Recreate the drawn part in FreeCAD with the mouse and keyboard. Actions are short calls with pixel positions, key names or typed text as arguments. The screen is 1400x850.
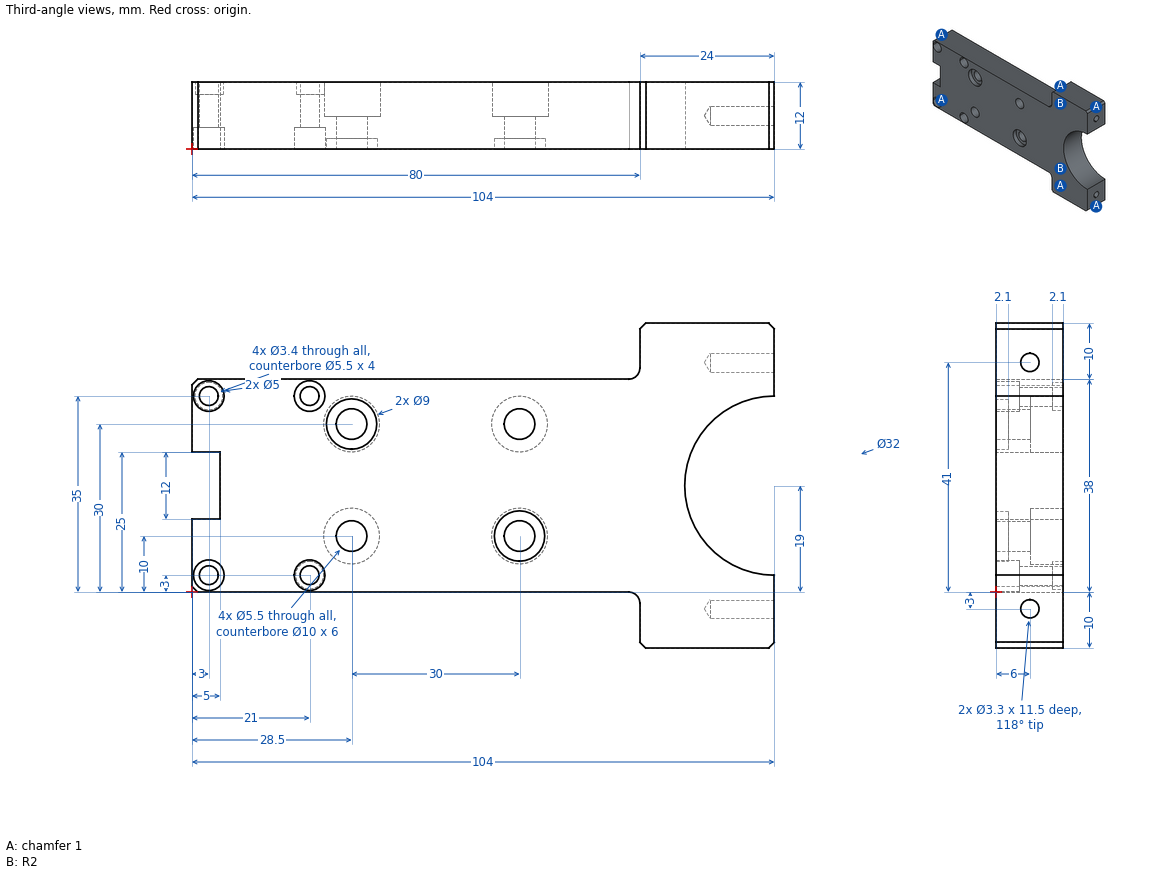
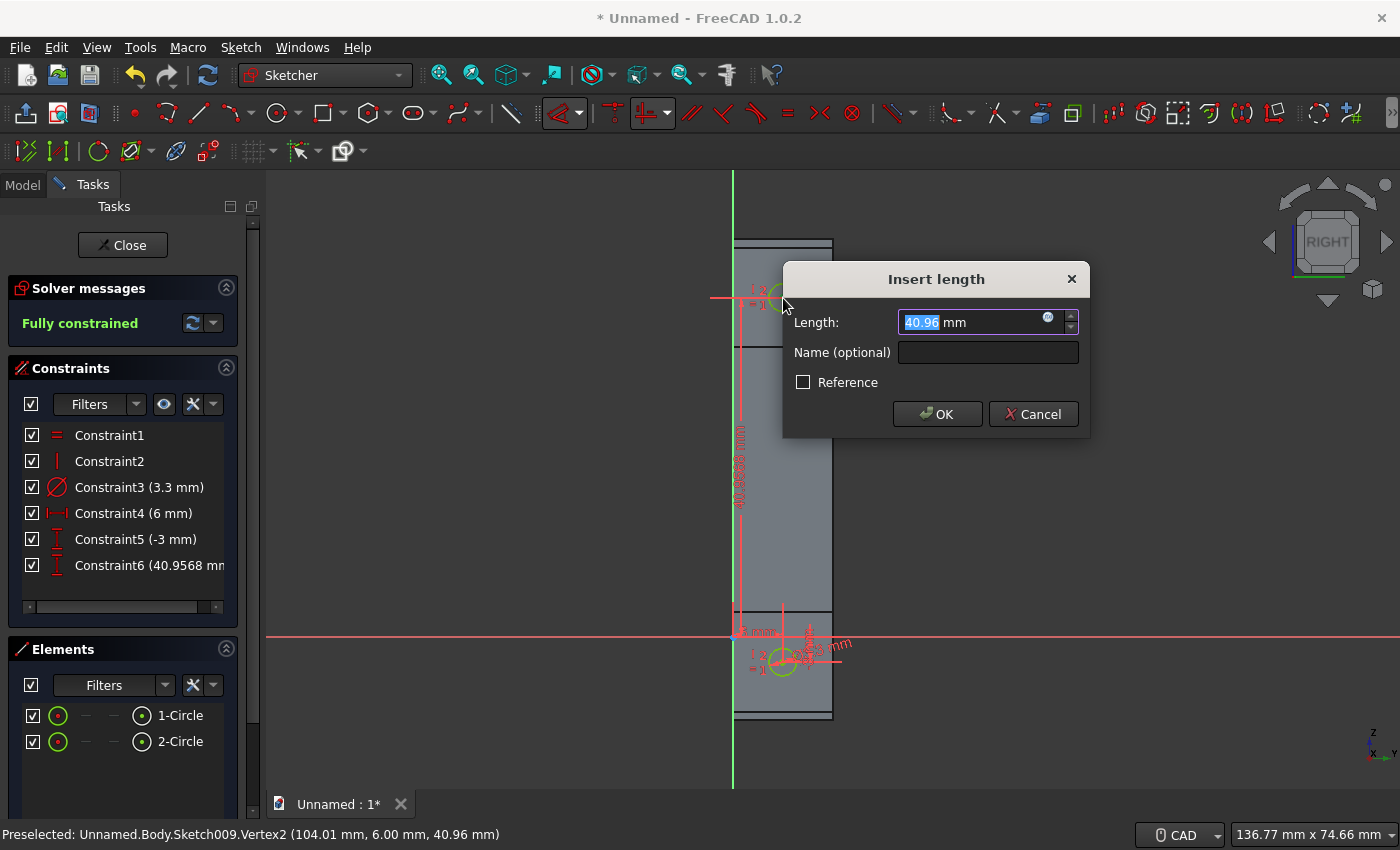
text(41)
key(Return)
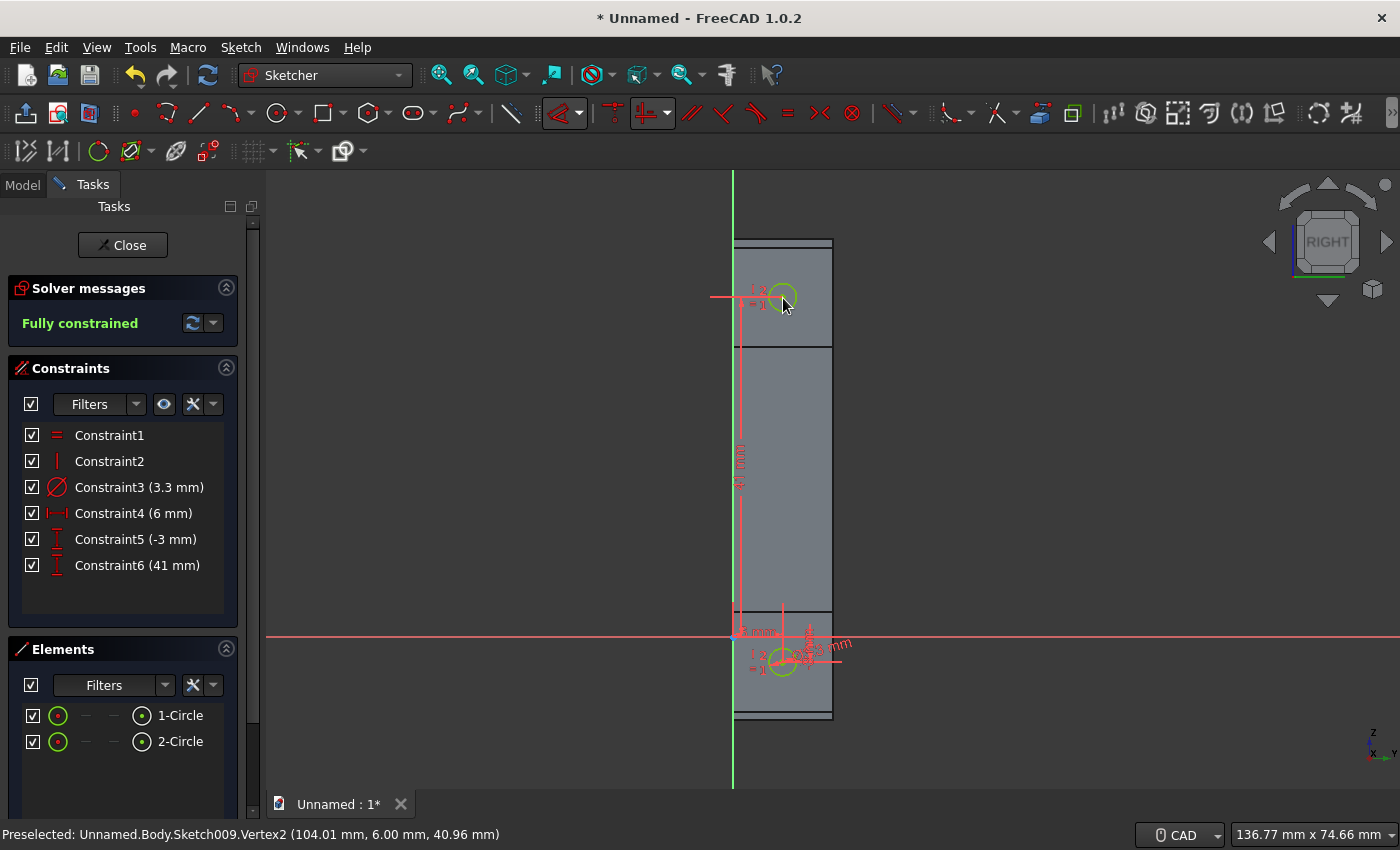
click(123, 245)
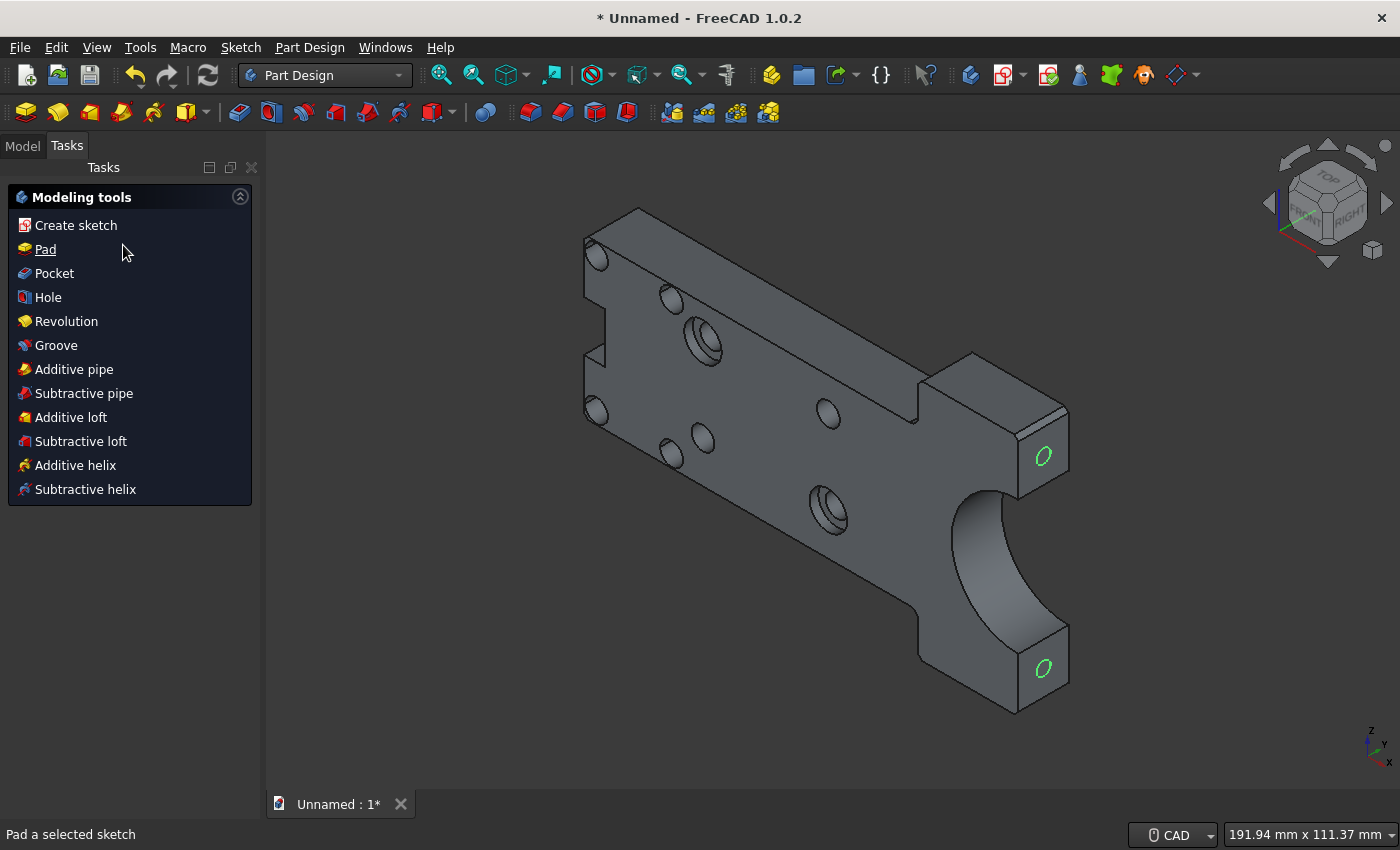
click(272, 112)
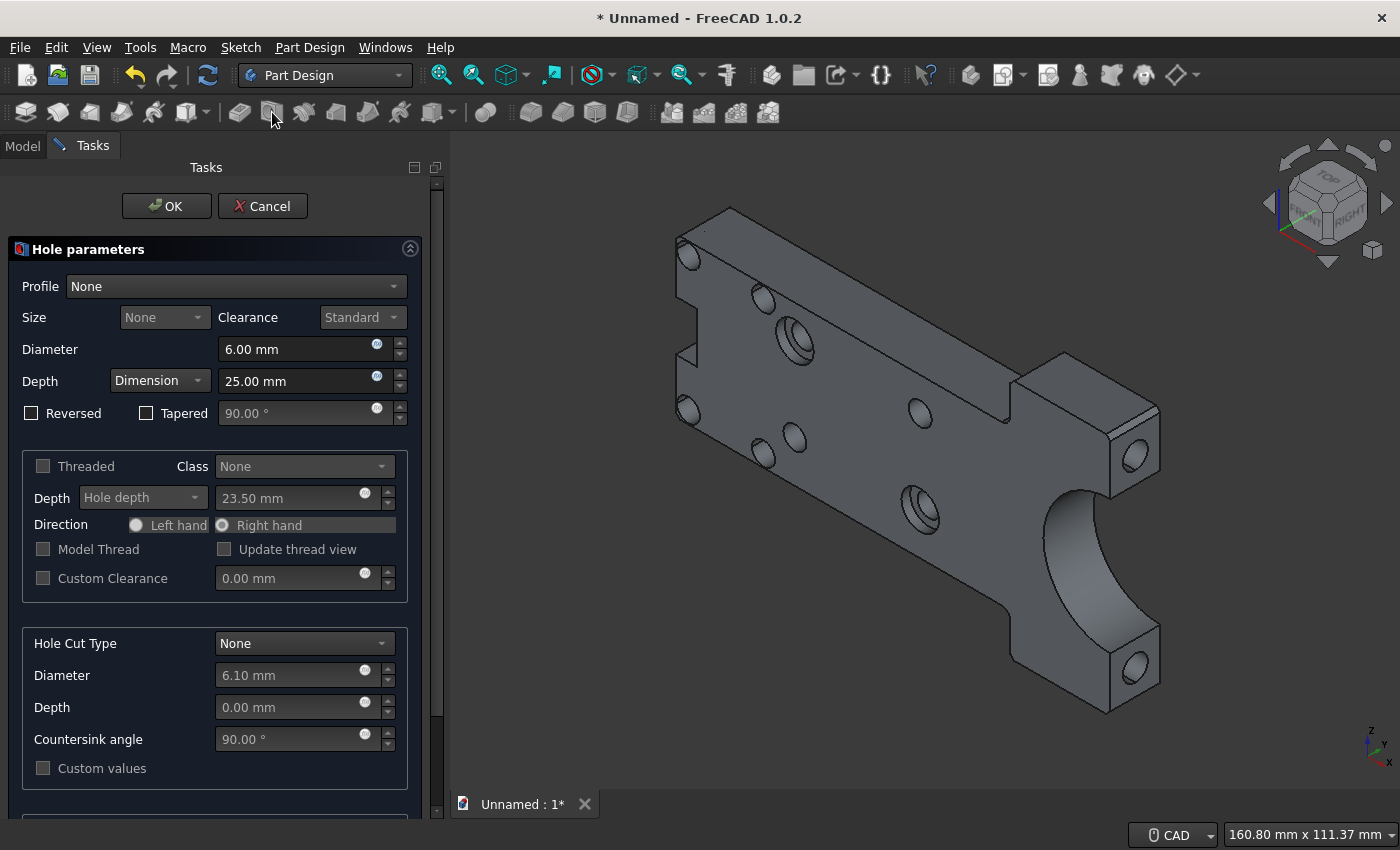
triple_click(305, 349)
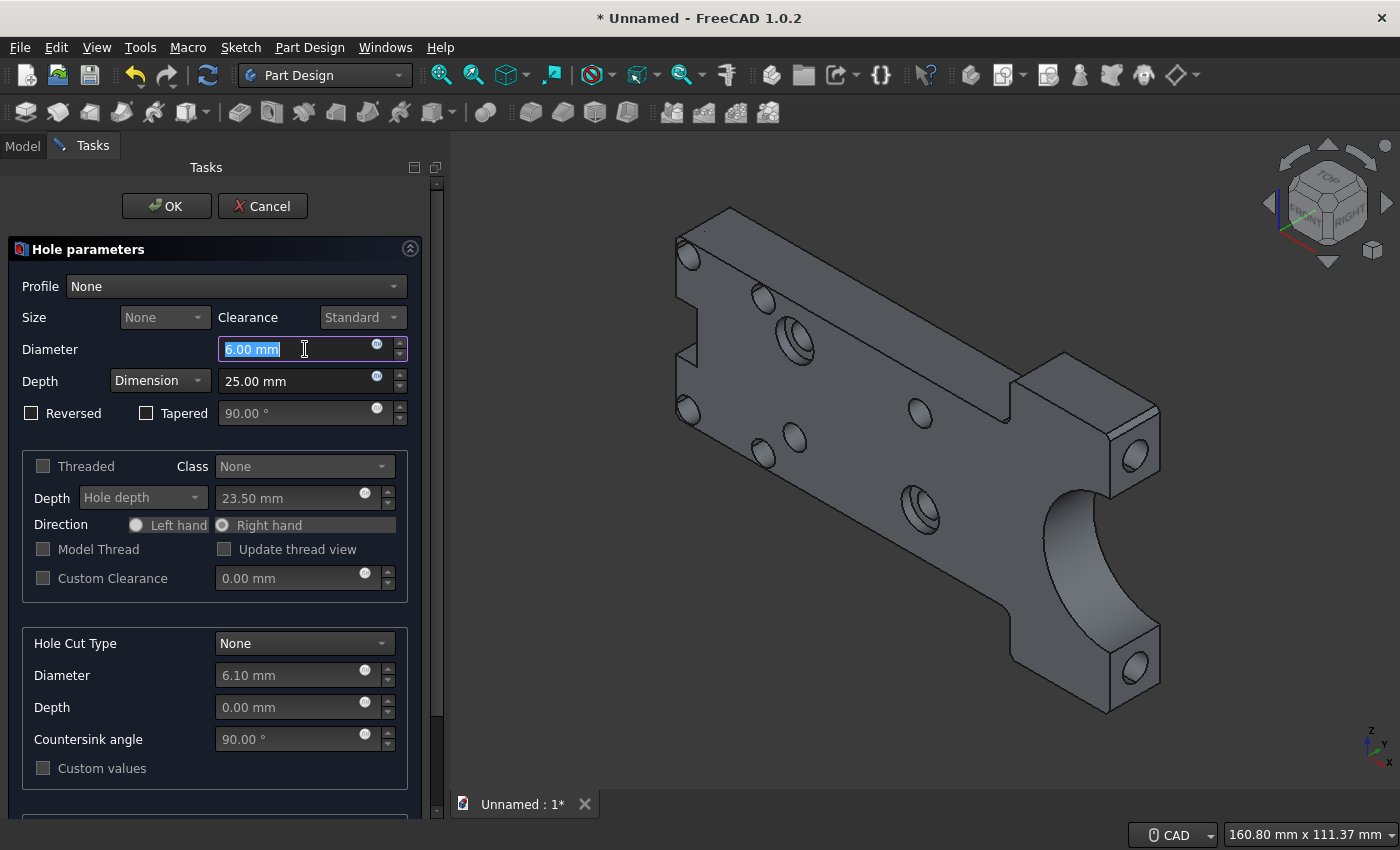
text(3.3)
key(Tab)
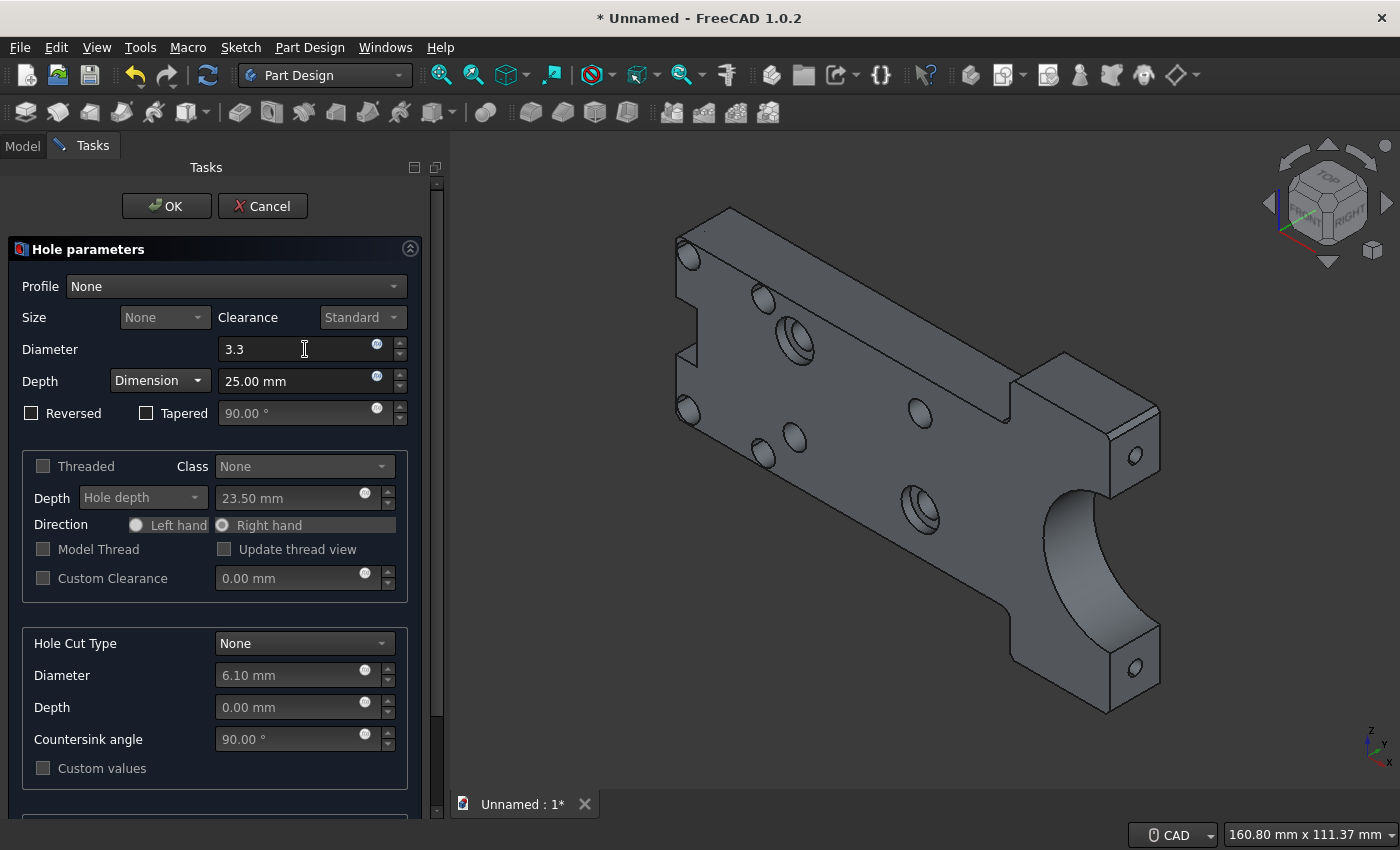
triple_click(305, 381)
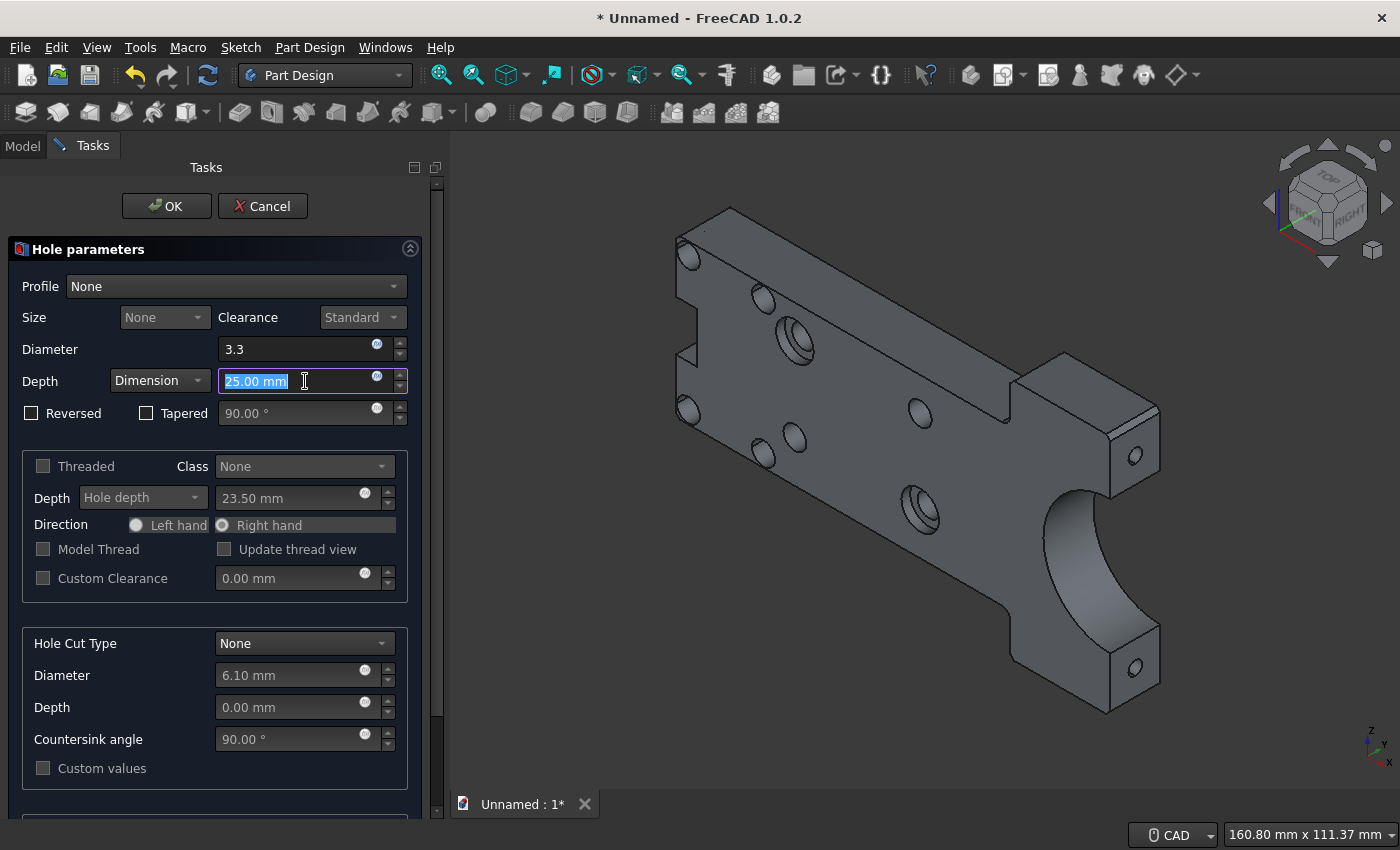
text(11.5)
key(Tab)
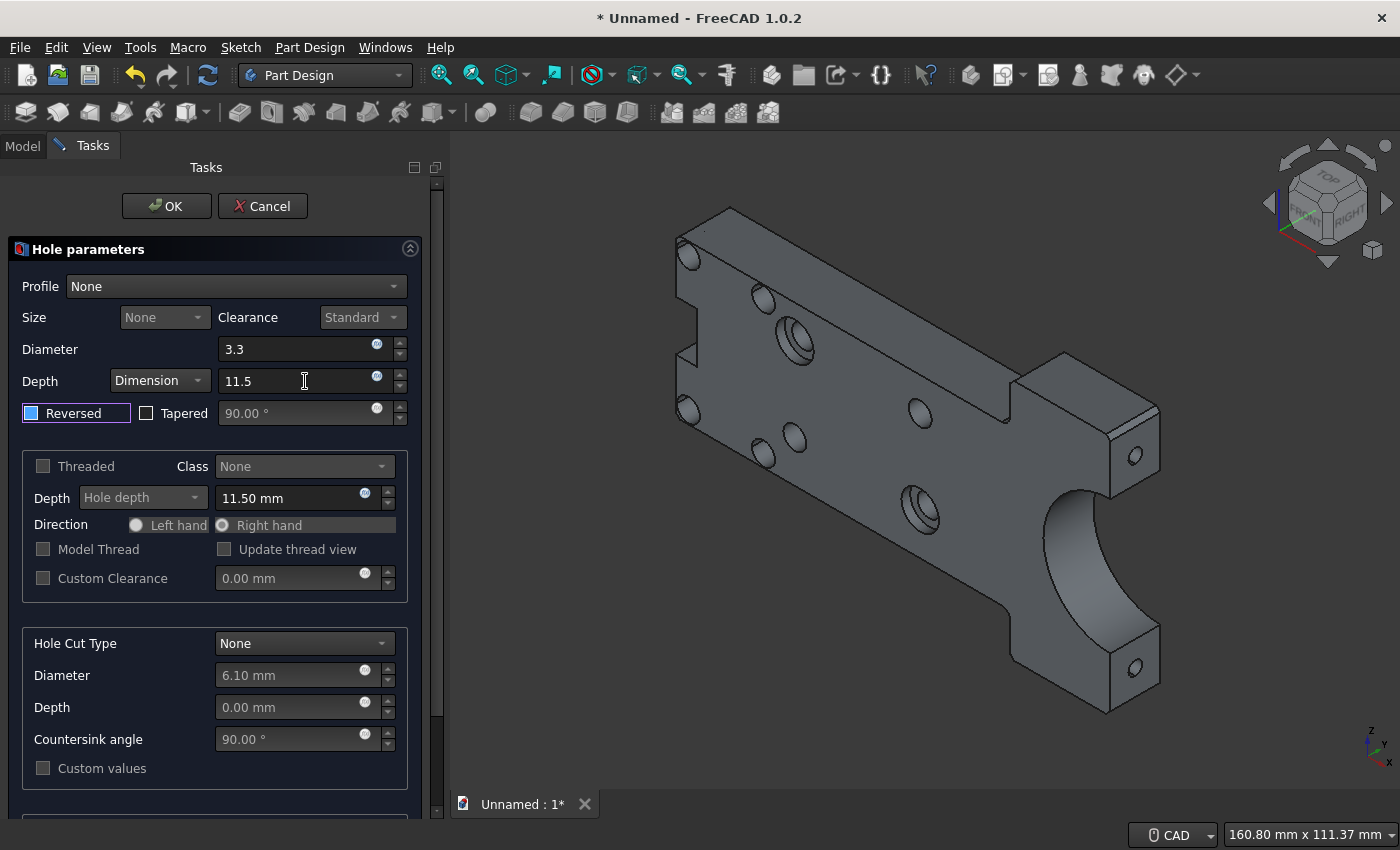
click(167, 206)